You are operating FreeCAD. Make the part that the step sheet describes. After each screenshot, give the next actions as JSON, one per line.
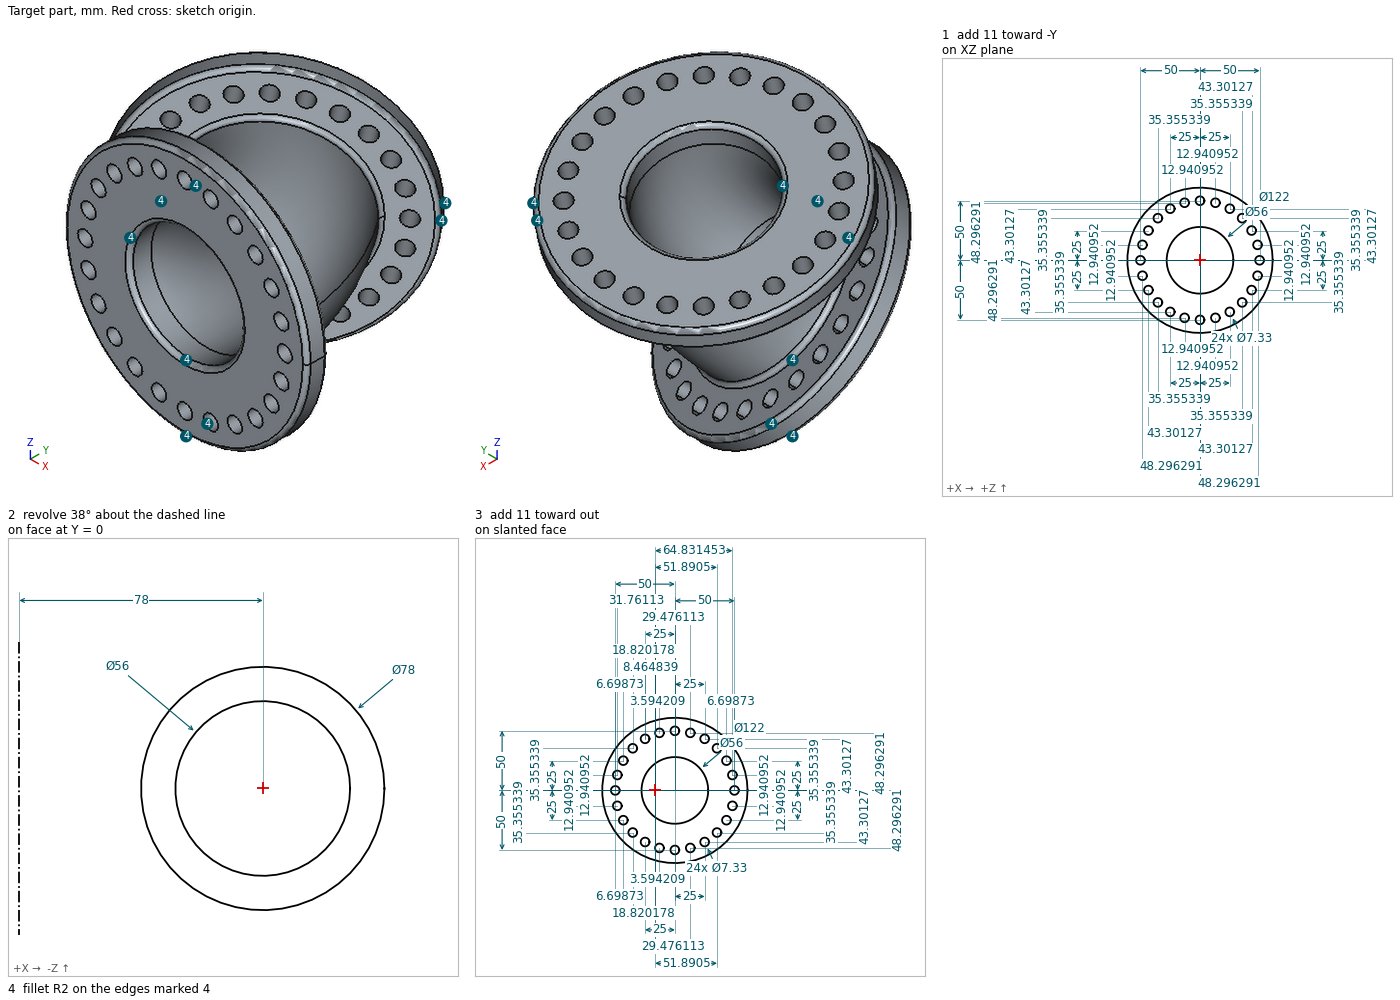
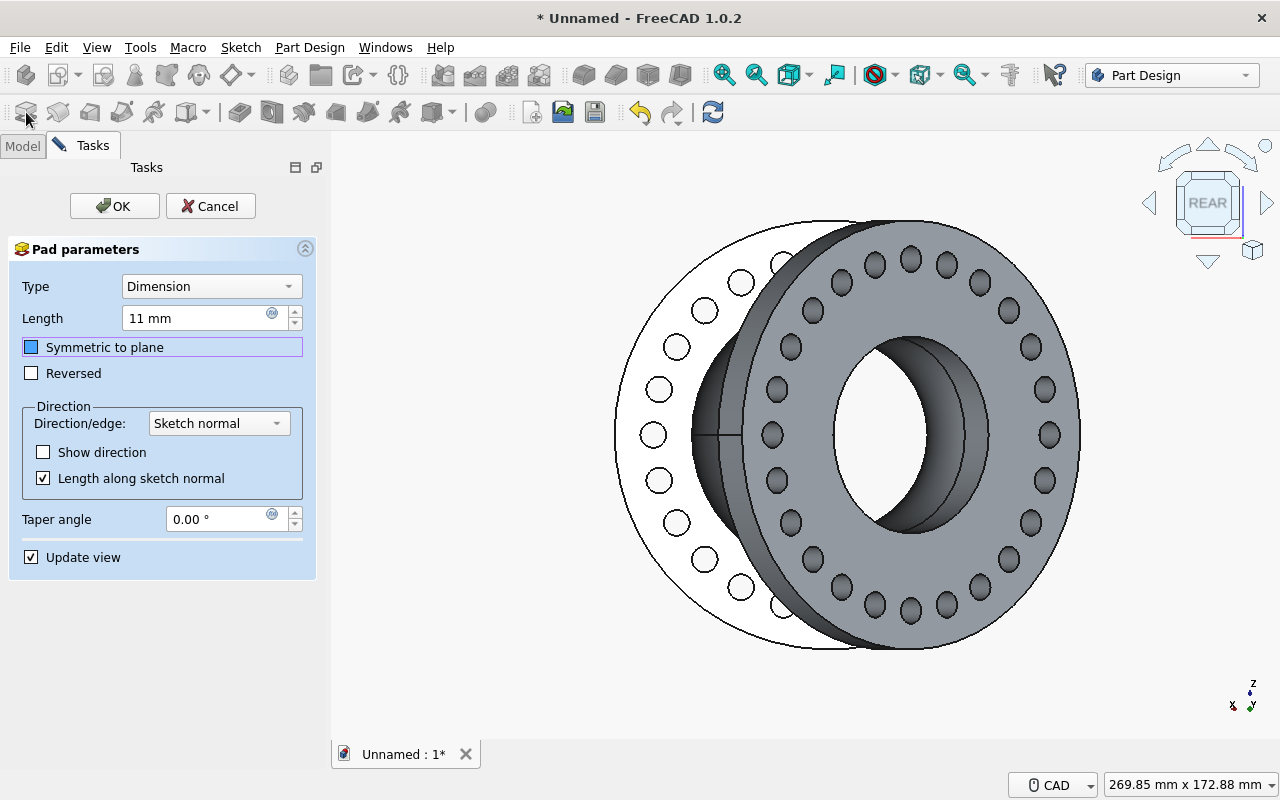
{"action": "left_click", "coordinate": [115, 206]}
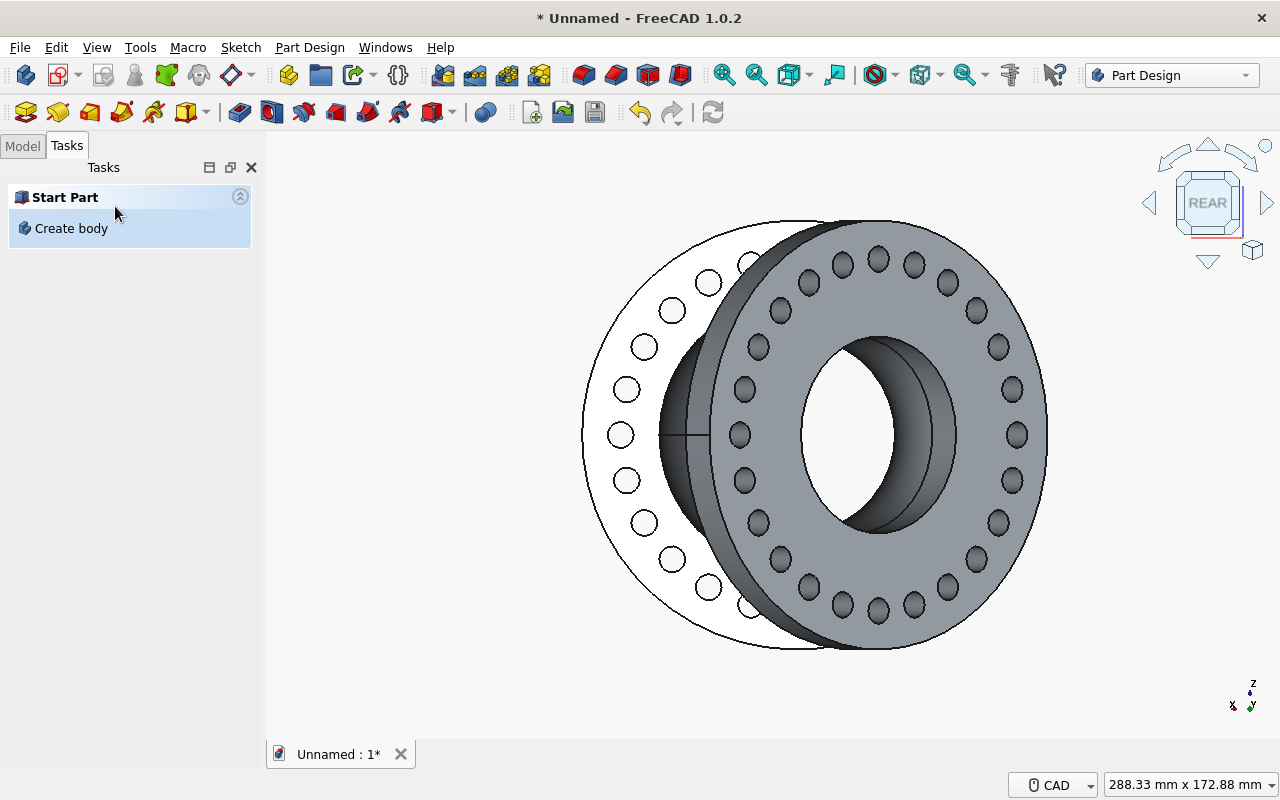
{"action": "left_click", "coordinate": [826, 638]}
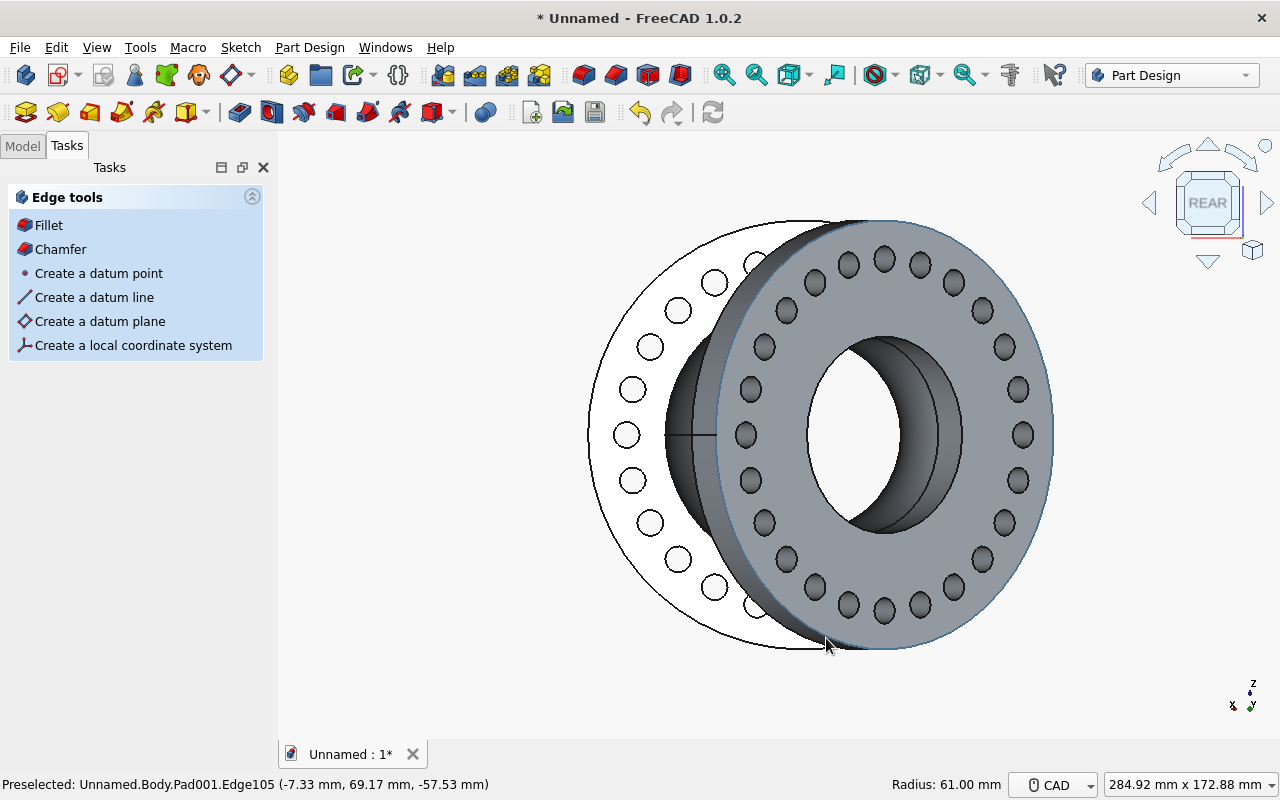
{"action": "left_click", "coordinate": [962, 434], "text": "ctrl"}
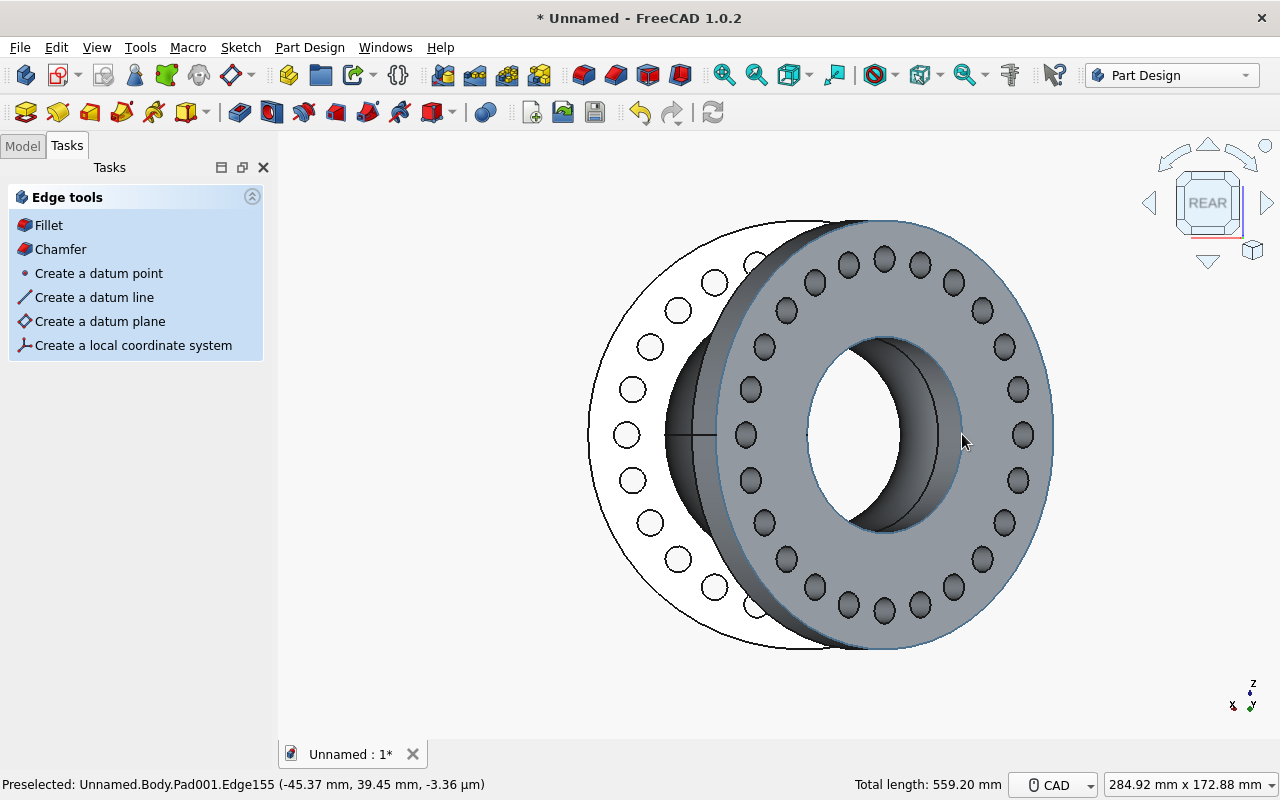
{"action": "left_click", "coordinate": [736, 638], "text": "ctrl"}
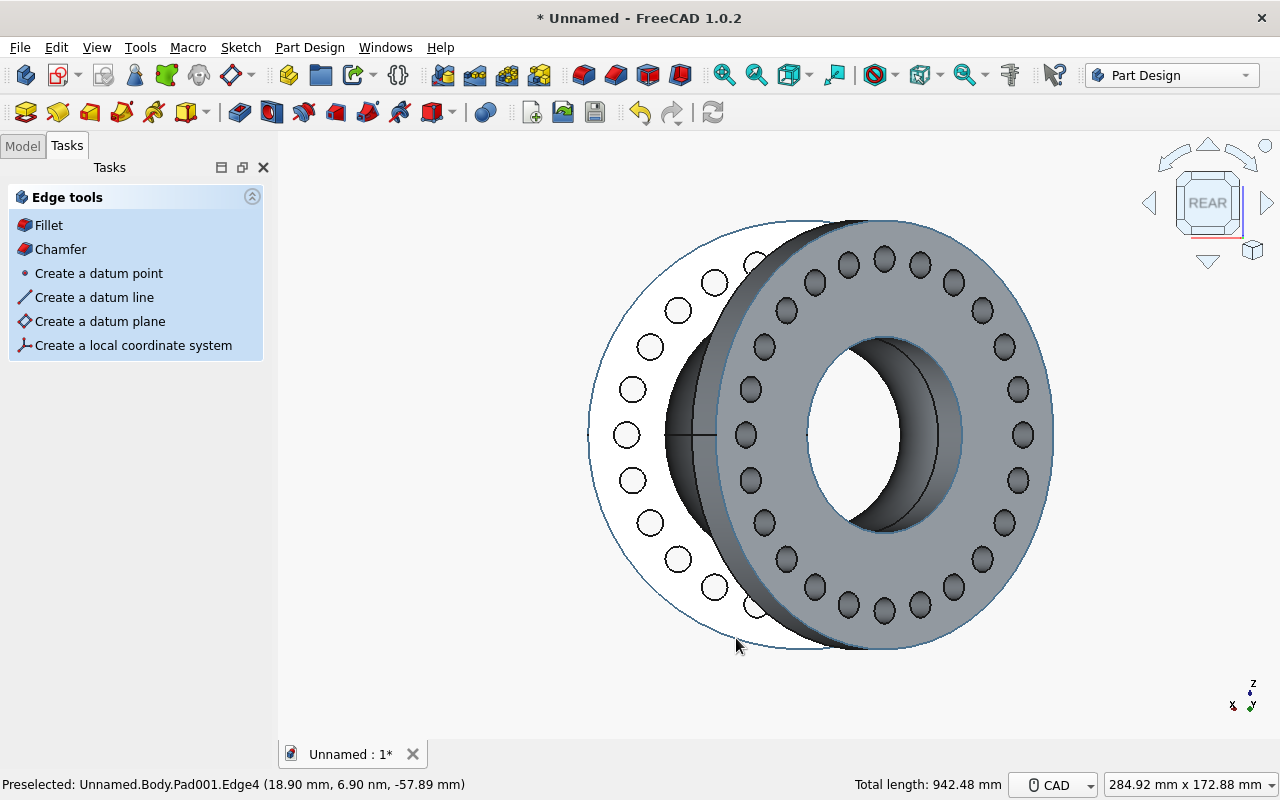
{"action": "key", "text": "0"}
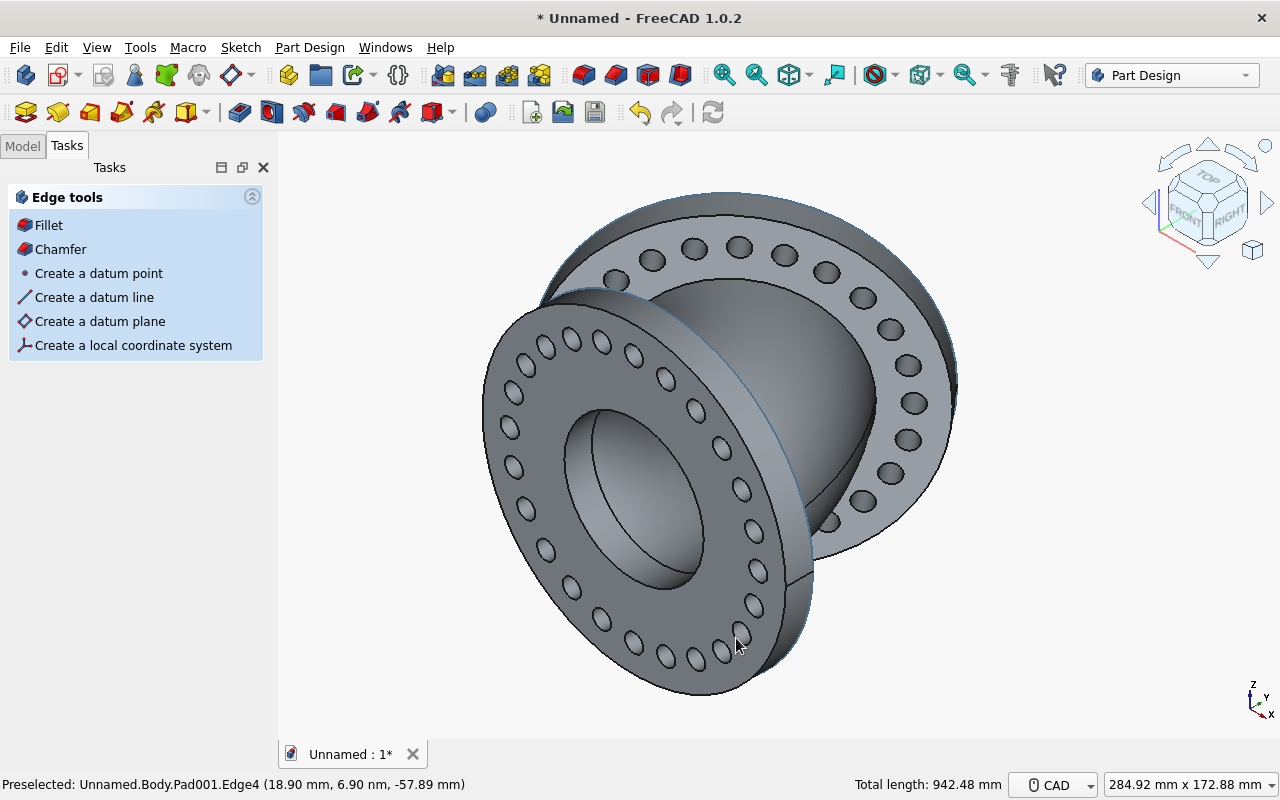
{"action": "left_click", "coordinate": [726, 76]}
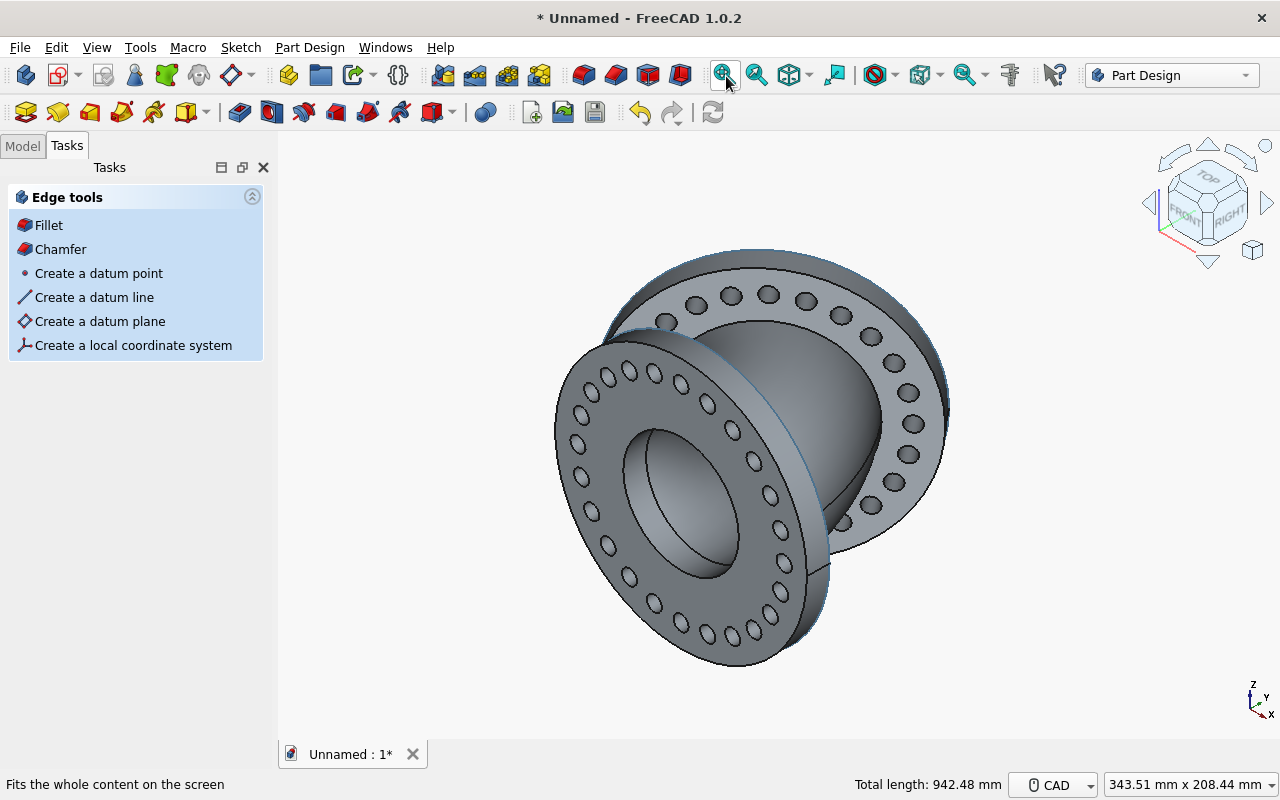
{"action": "left_click", "coordinate": [626, 317], "text": "ctrl"}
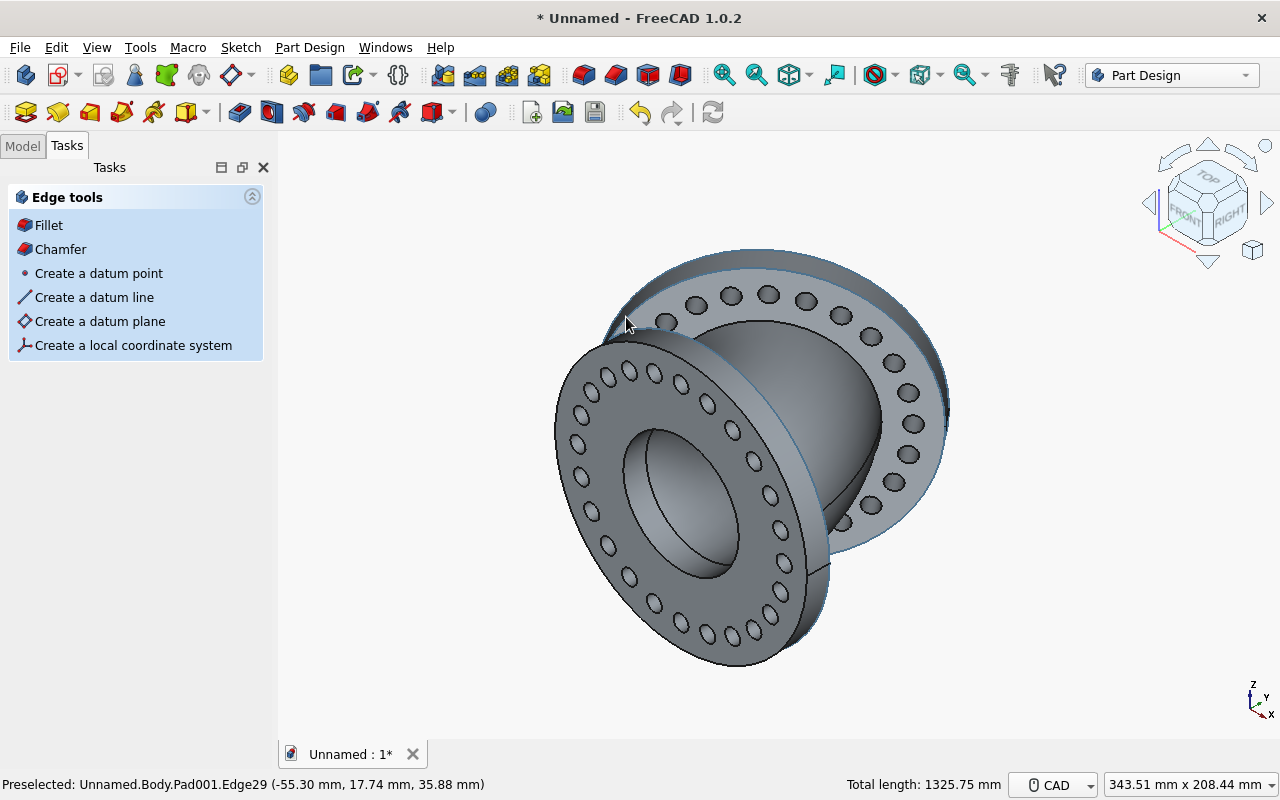
{"action": "left_click", "coordinate": [642, 342], "text": "ctrl"}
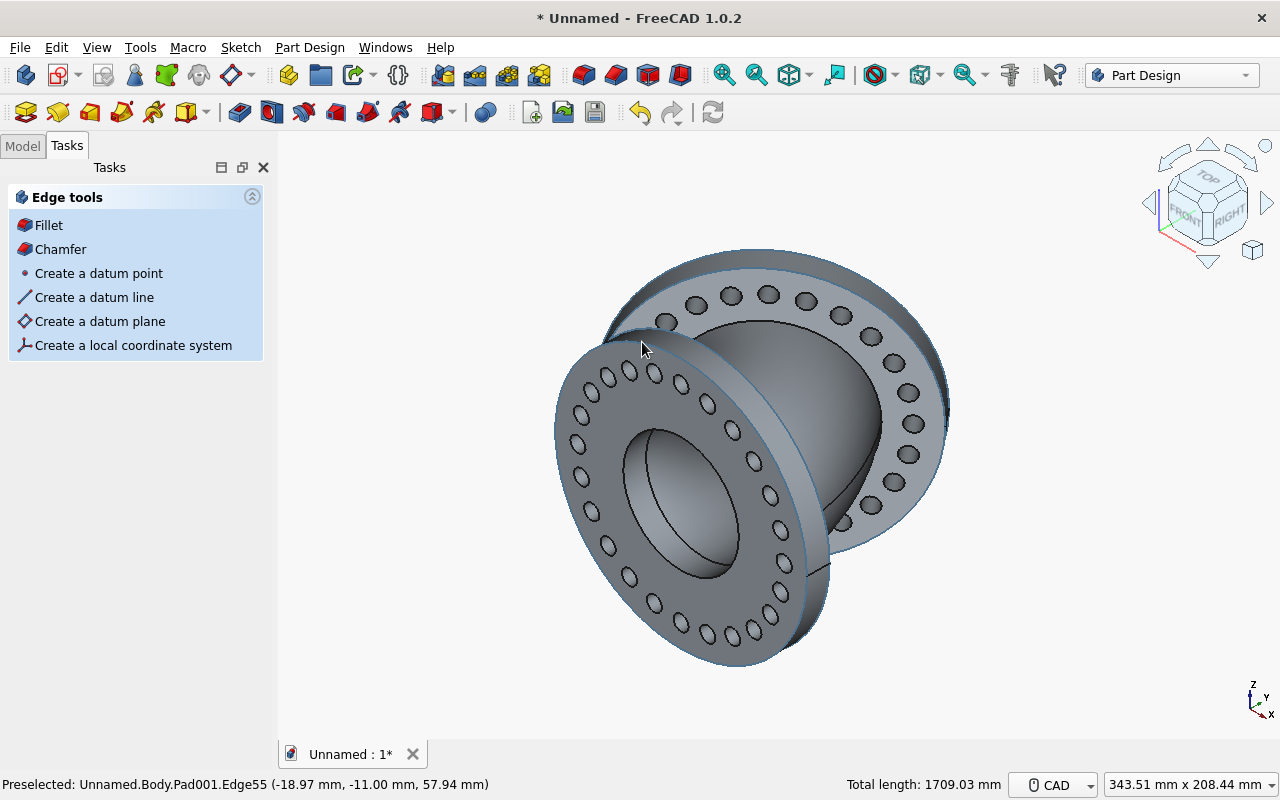
{"action": "left_click", "coordinate": [623, 469], "text": "ctrl"}